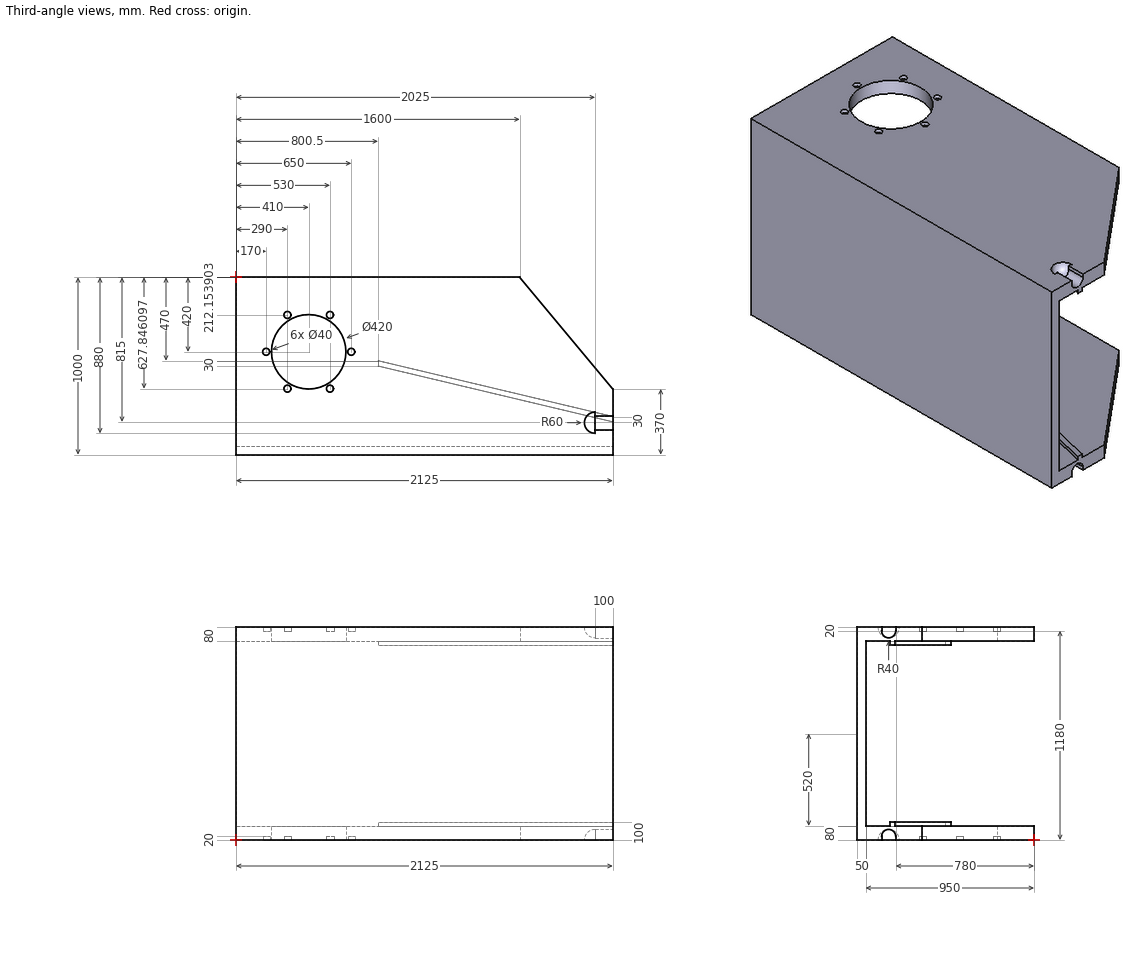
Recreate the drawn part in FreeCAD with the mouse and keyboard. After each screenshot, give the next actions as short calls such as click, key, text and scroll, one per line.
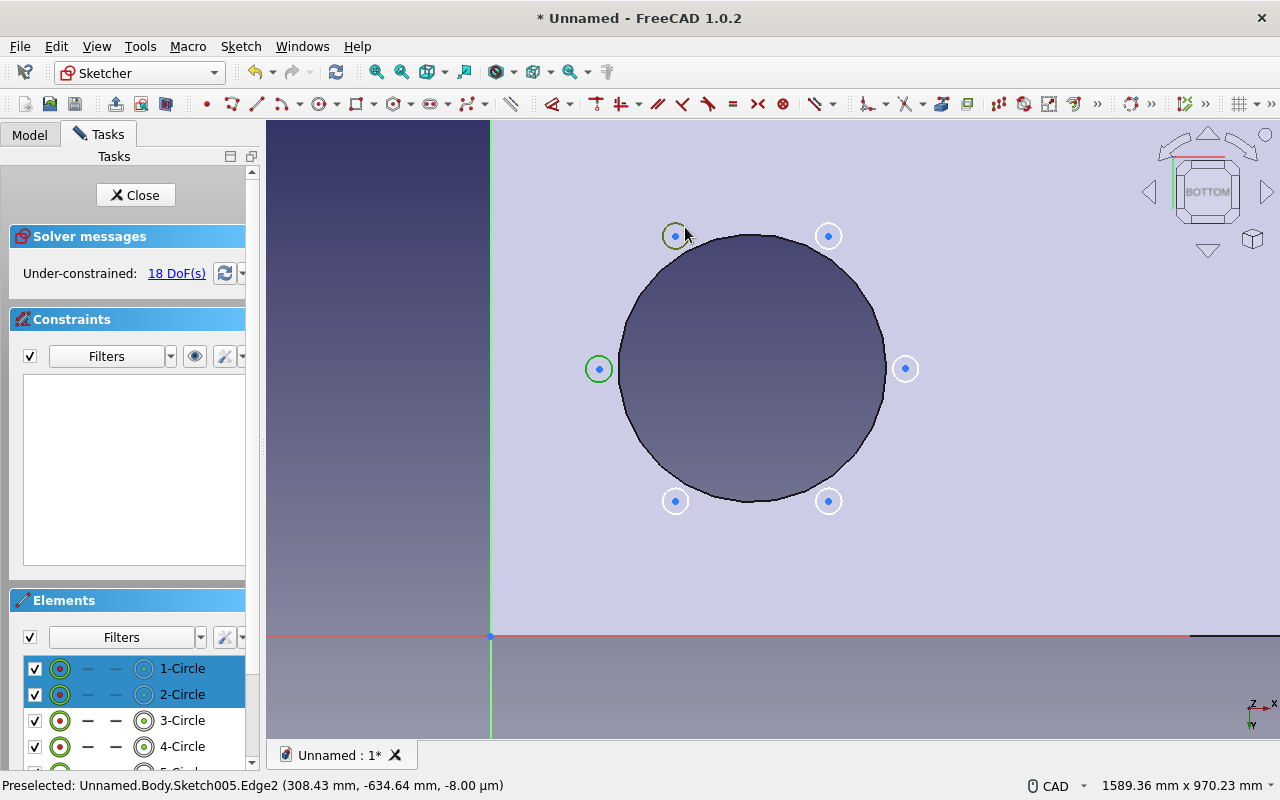
click(838, 227)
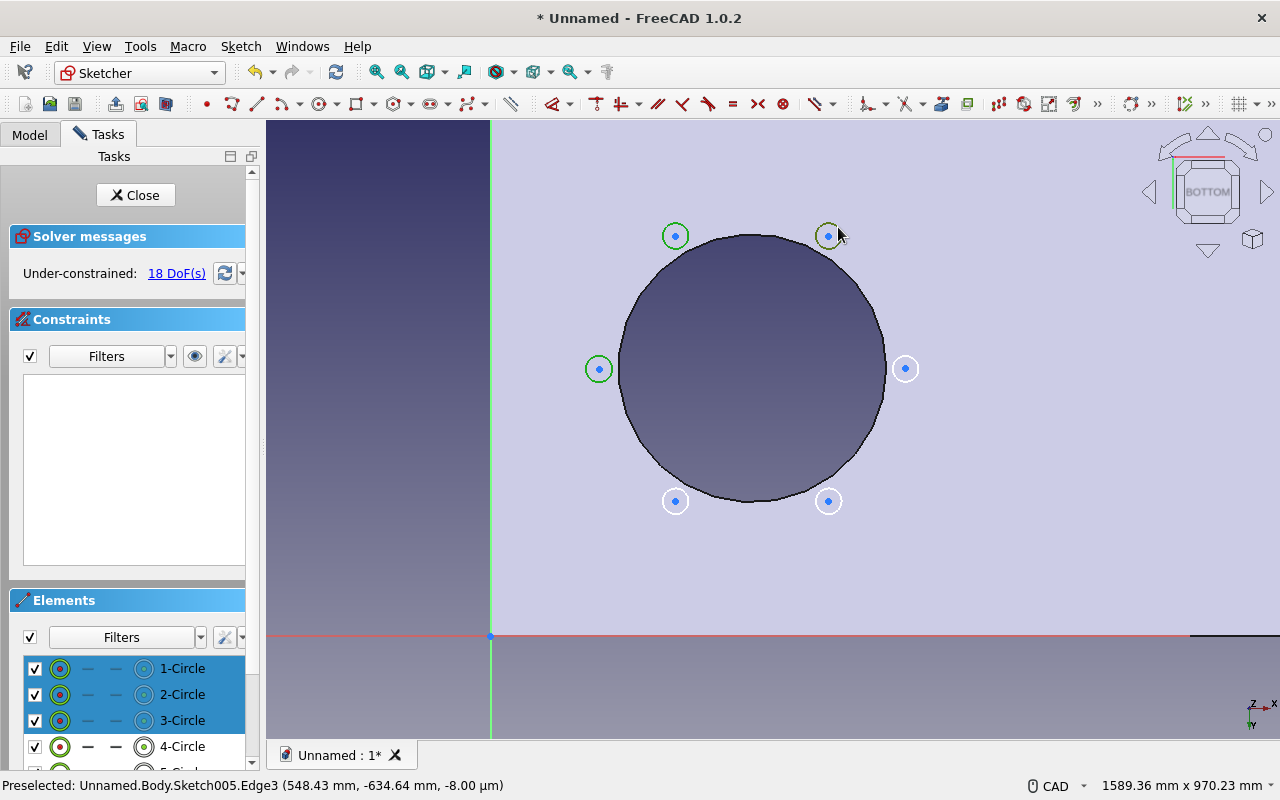
click(915, 360)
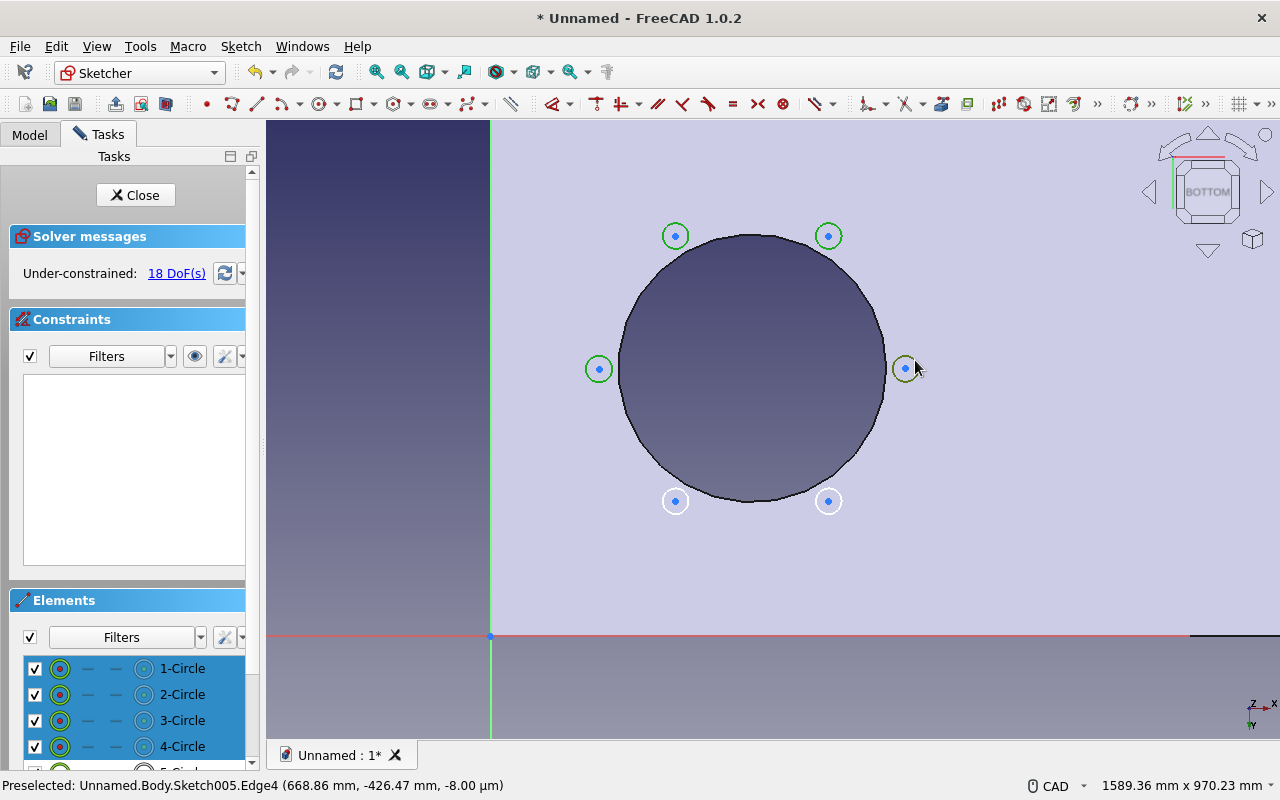
click(685, 492)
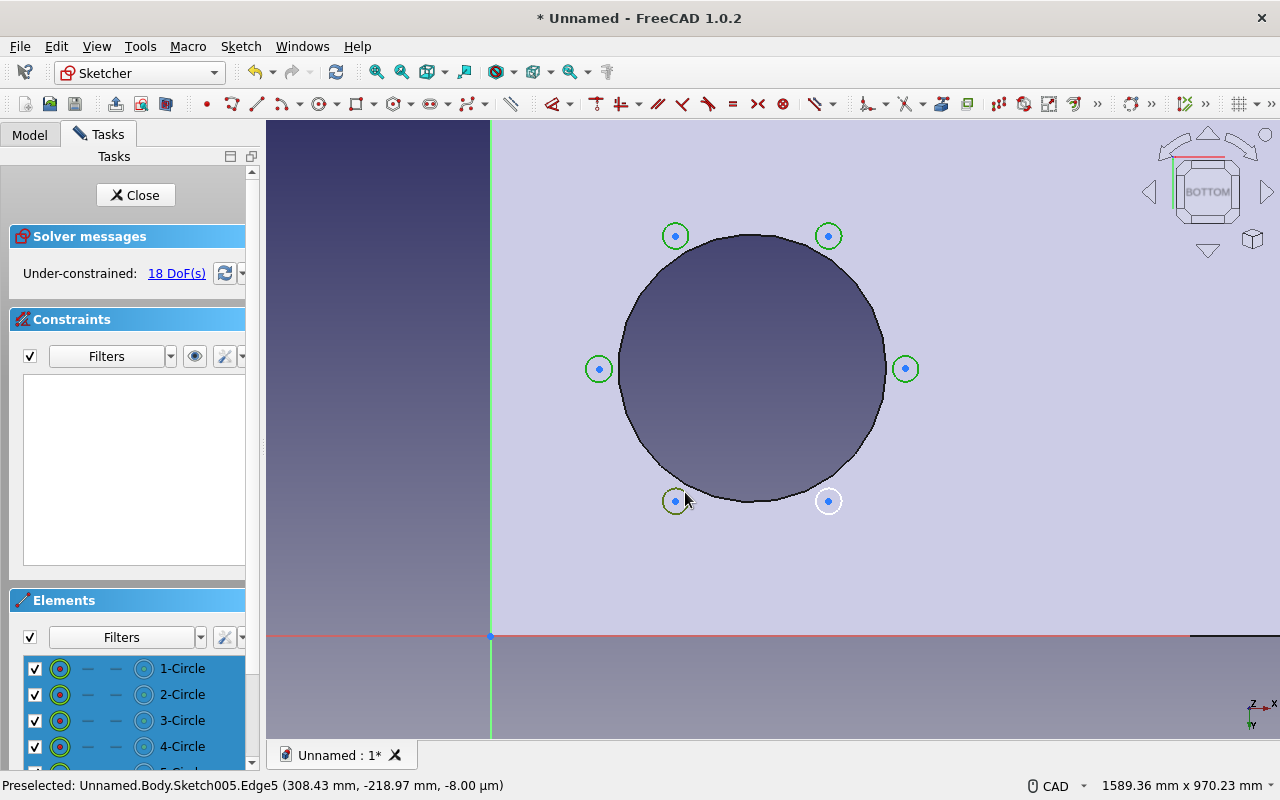
click(838, 492)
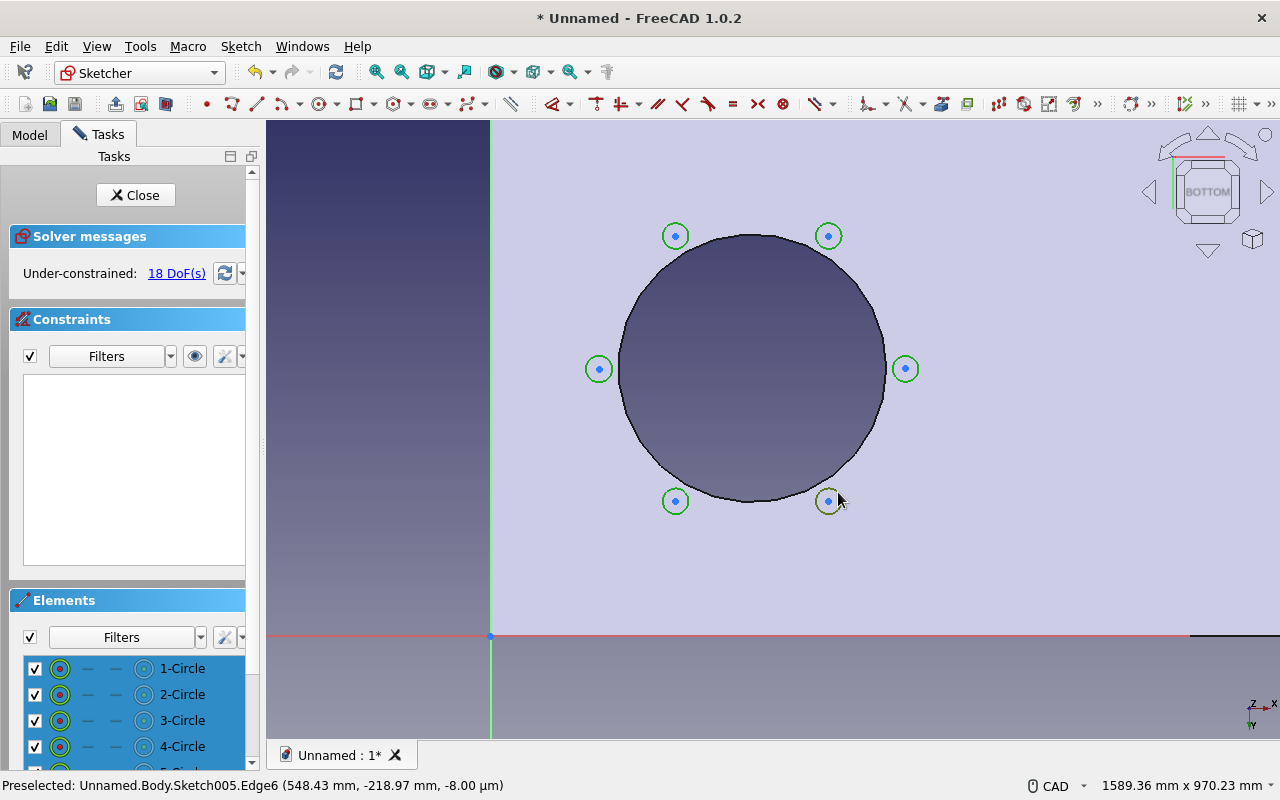
key(e)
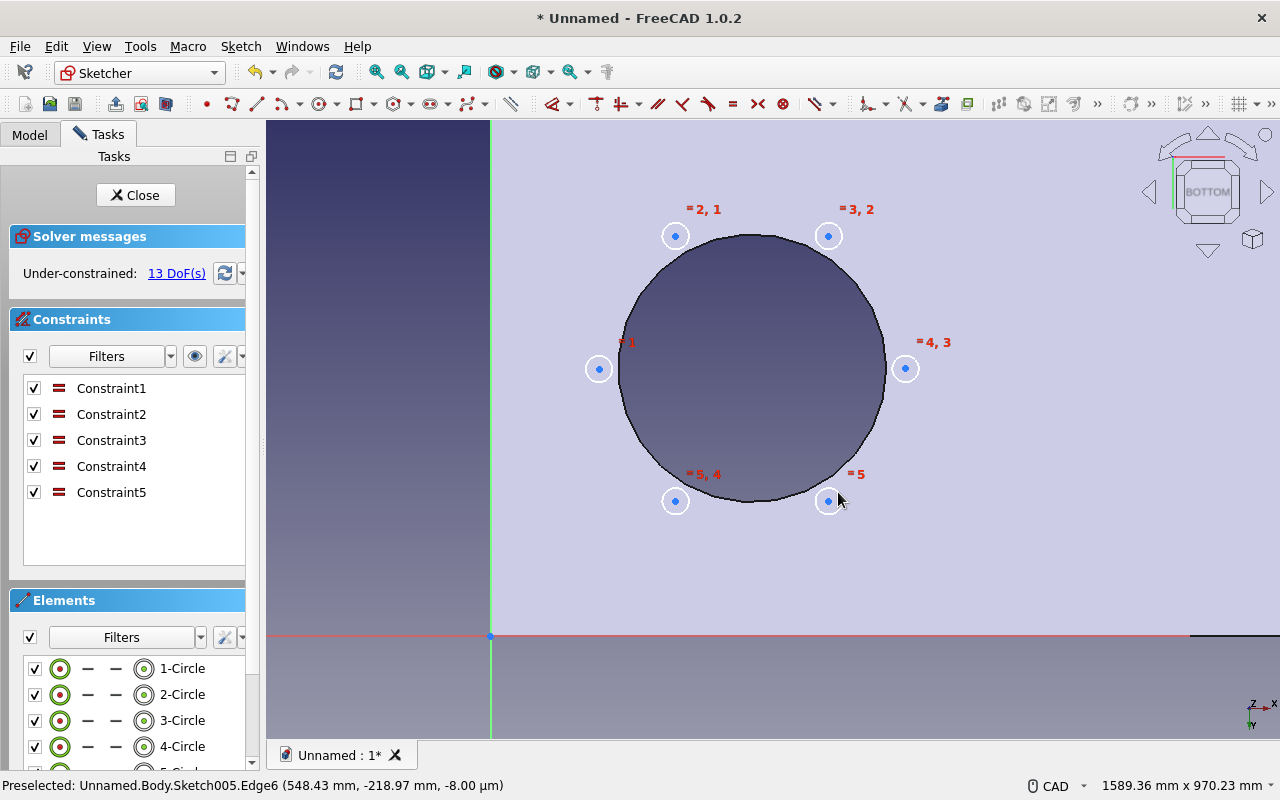
click(676, 236)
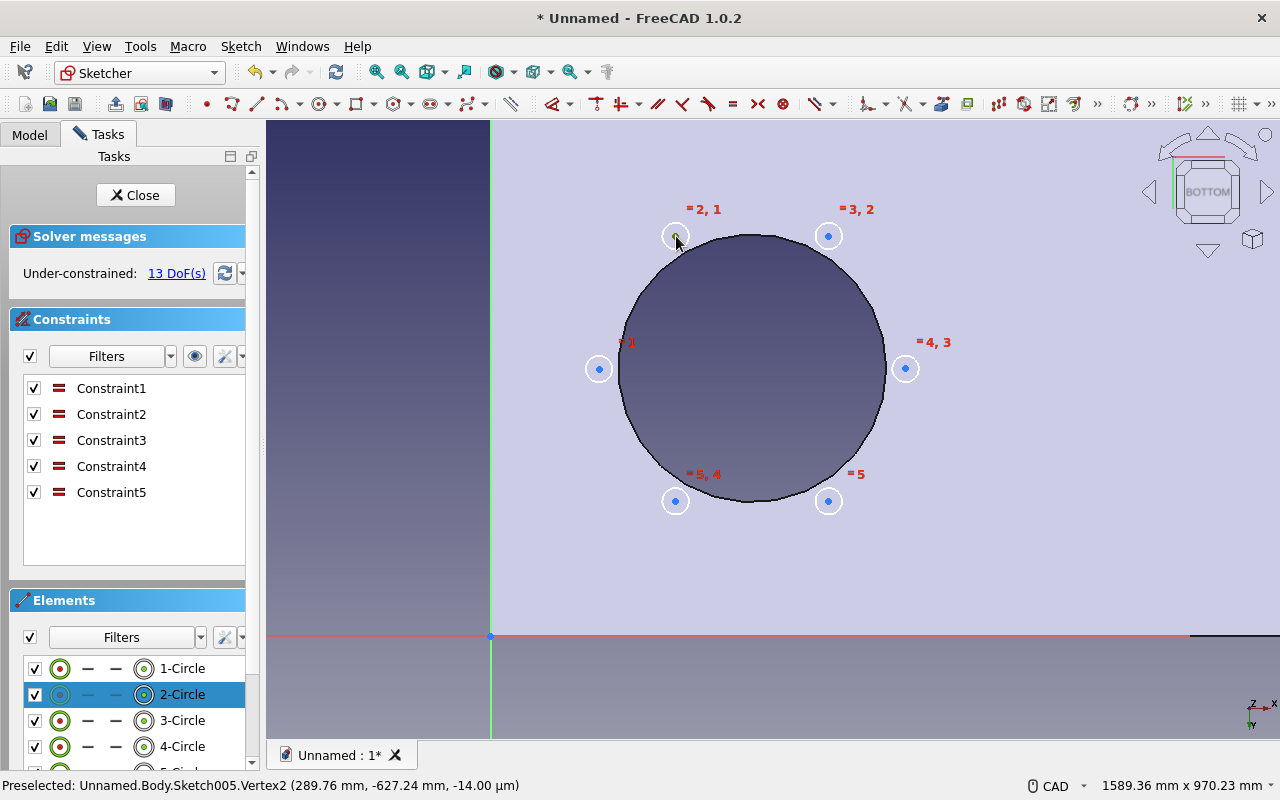
click(829, 236)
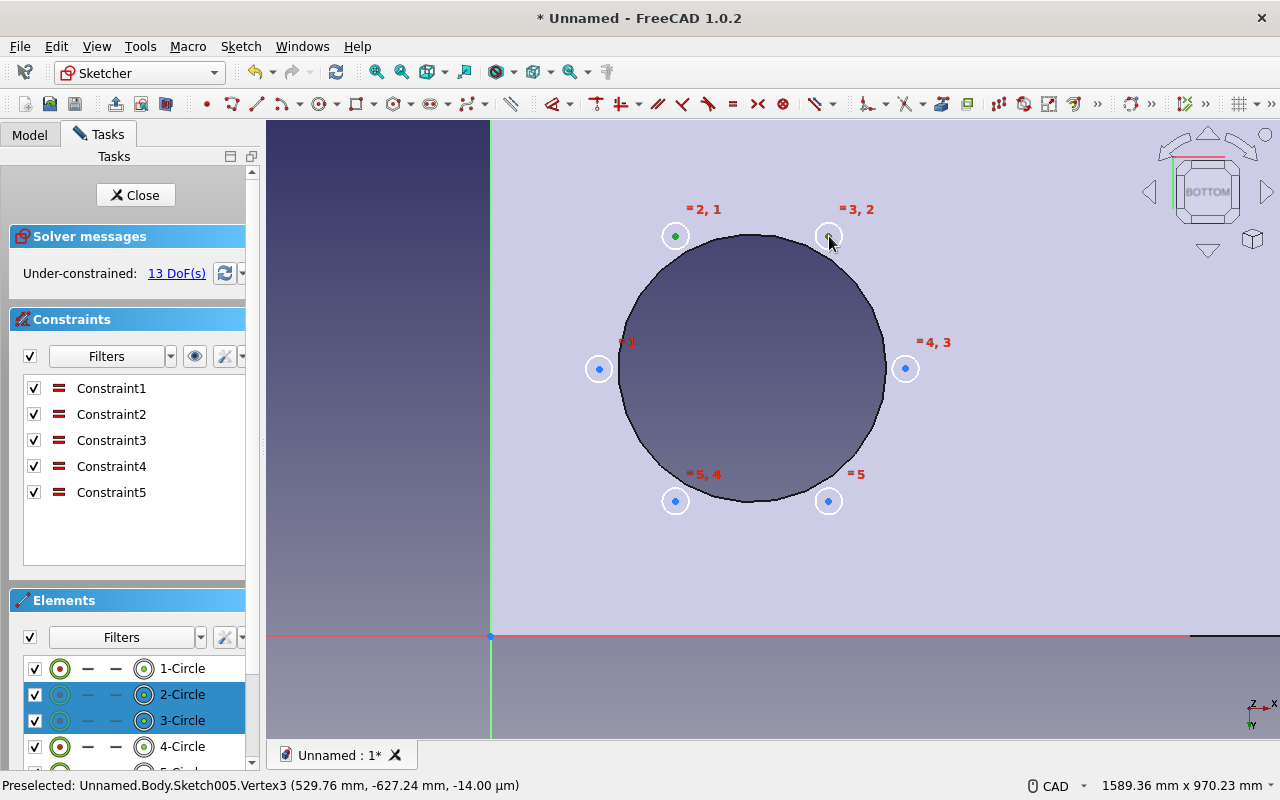
key(h)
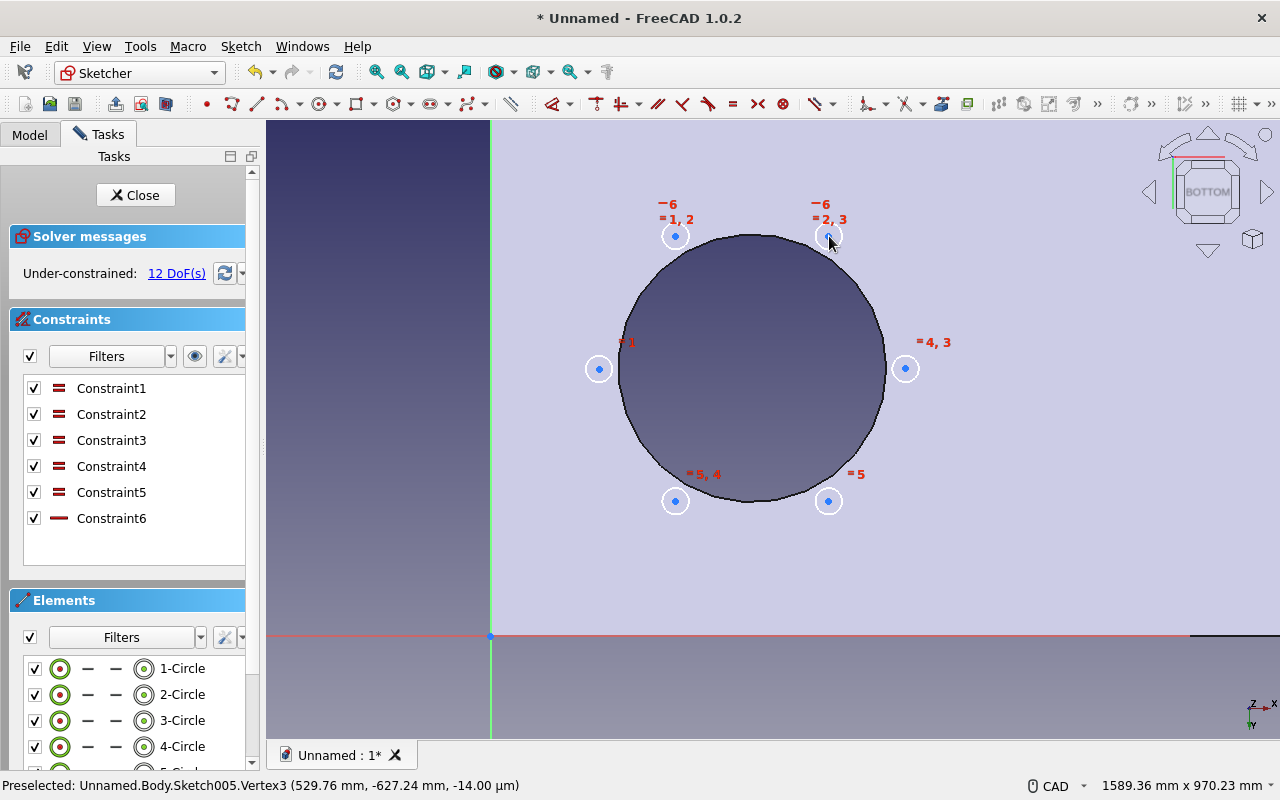
click(599, 369)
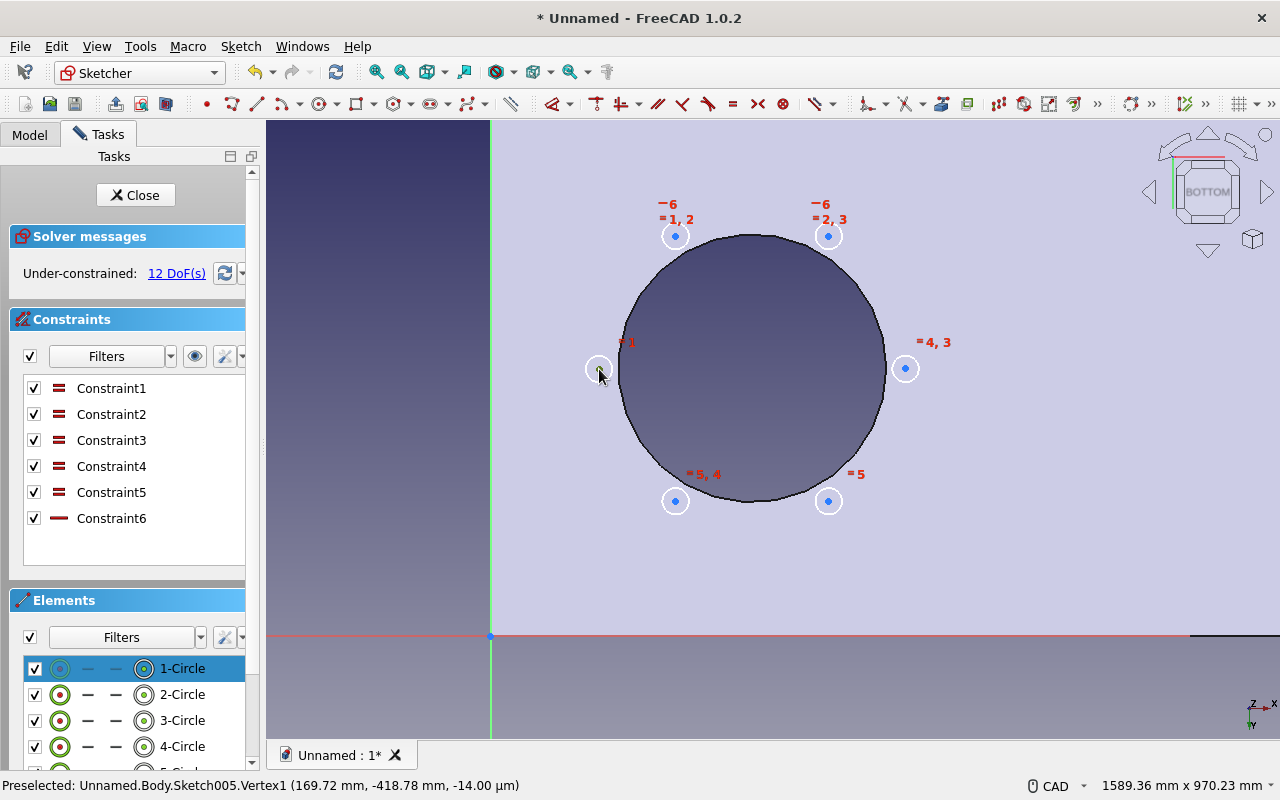
click(906, 369)